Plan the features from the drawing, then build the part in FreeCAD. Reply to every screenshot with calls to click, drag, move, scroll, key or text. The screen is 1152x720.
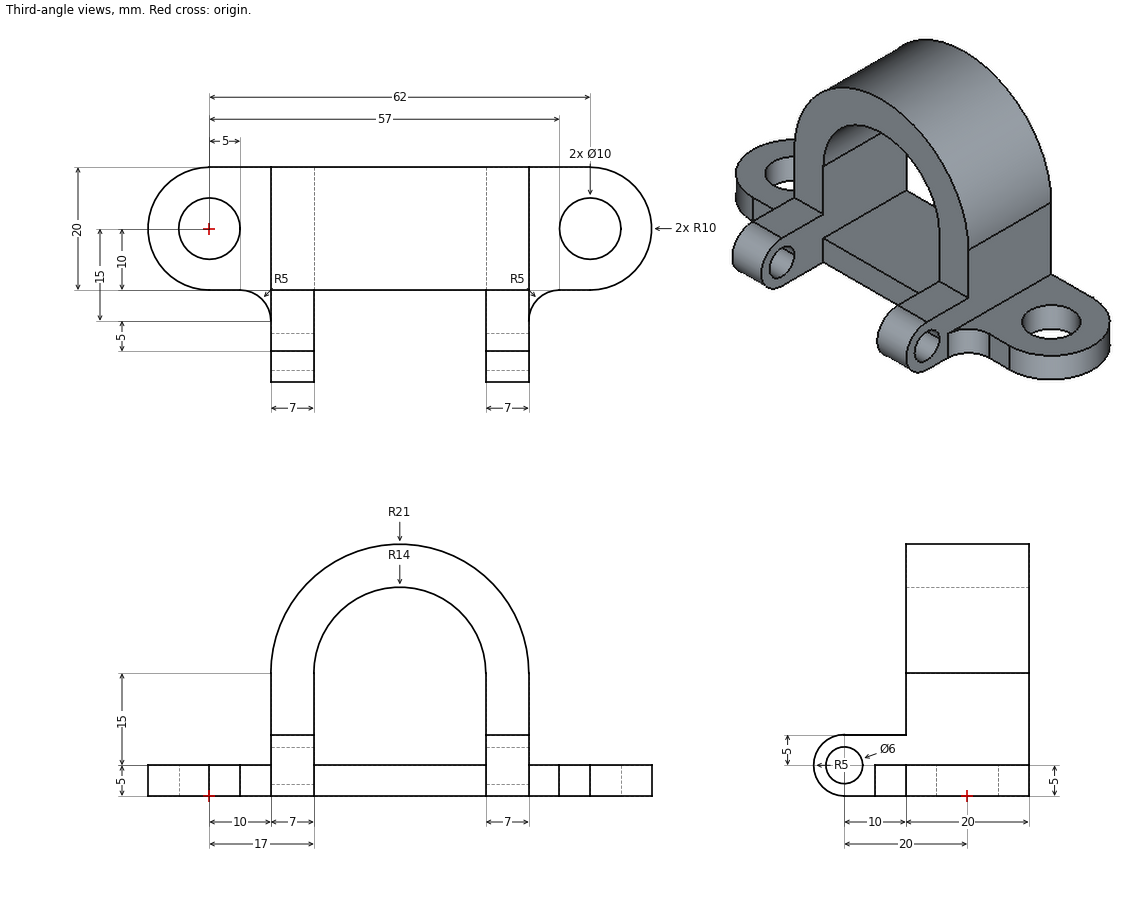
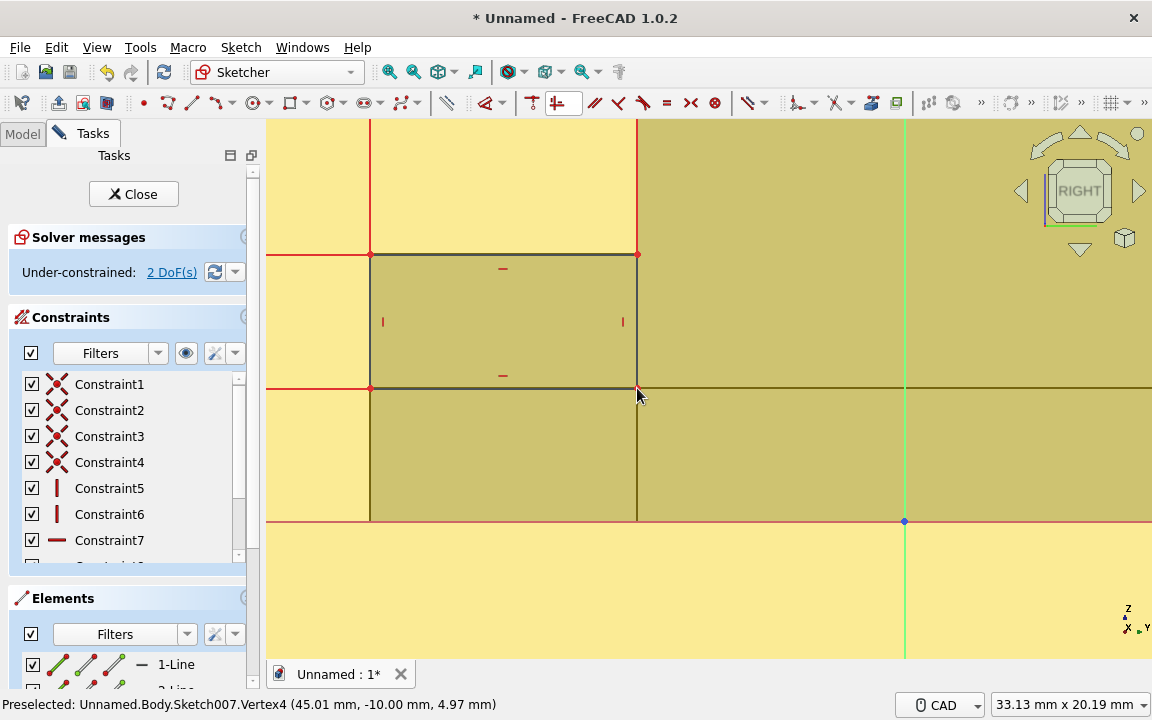
click(486, 104)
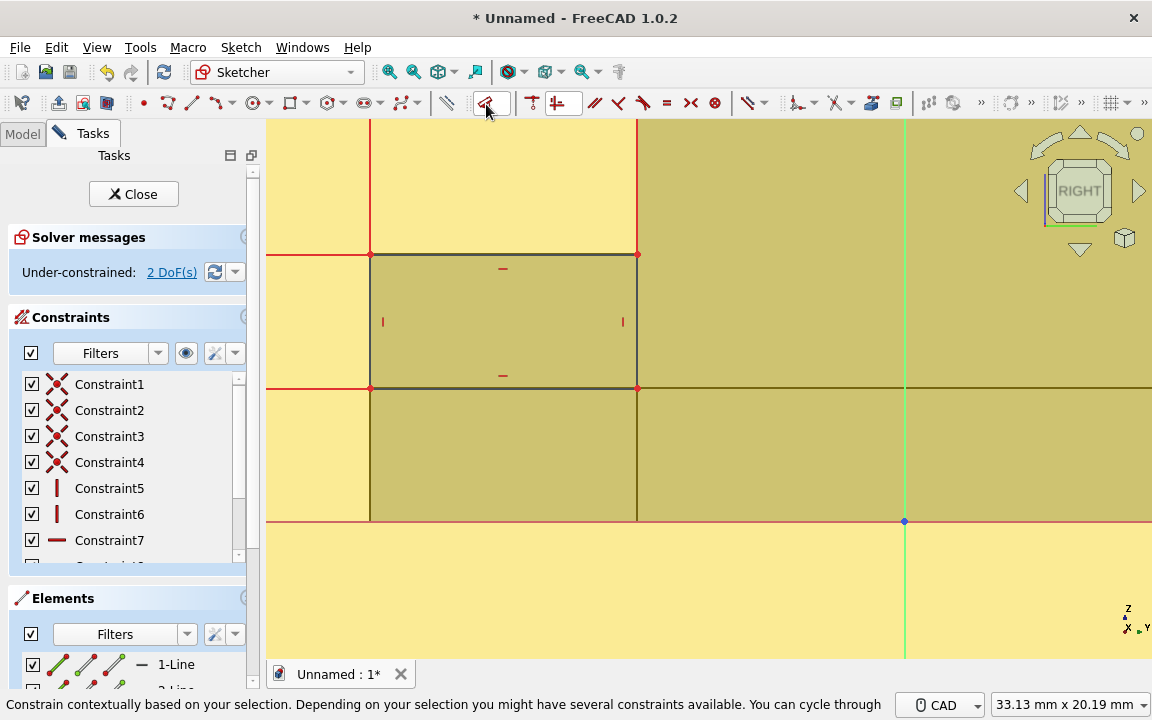
click(370, 389)
click(939, 455)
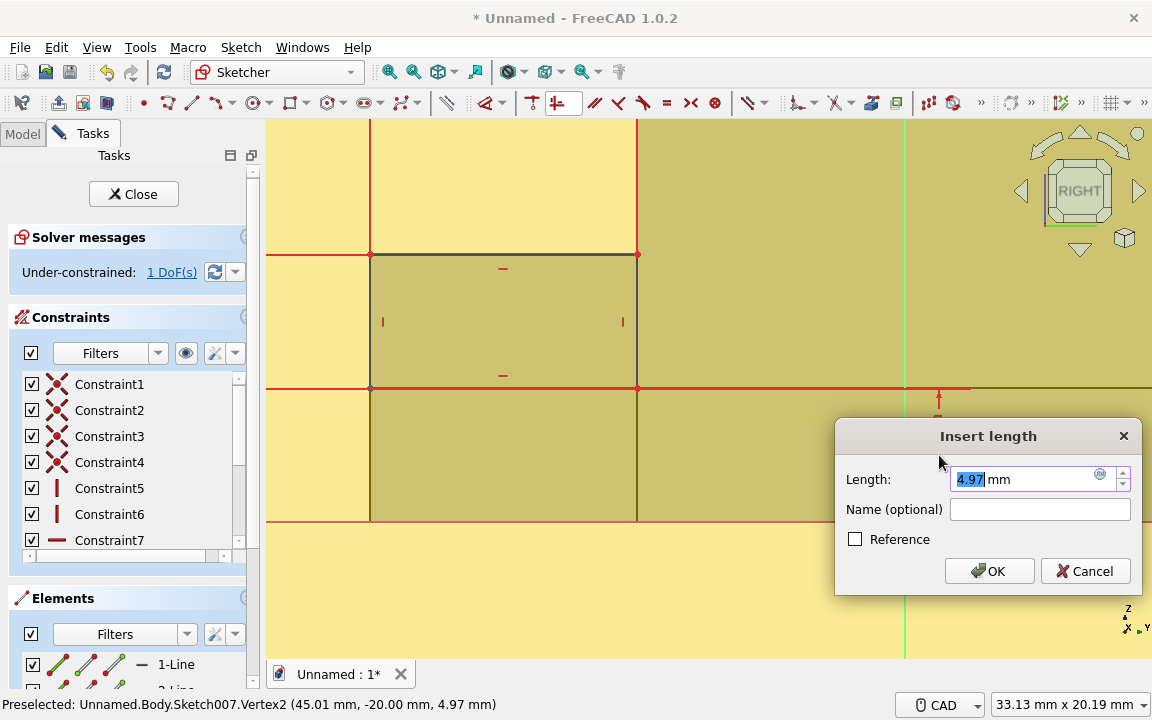
text(5)
key(Return)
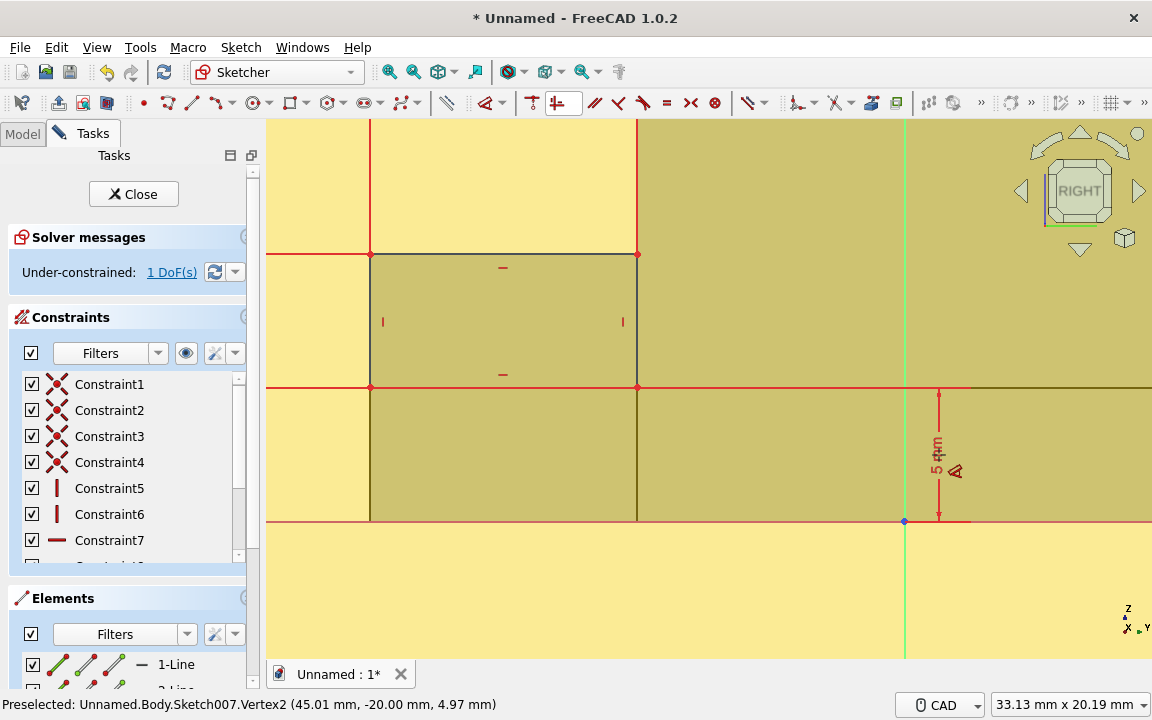
click(370, 254)
click(637, 556)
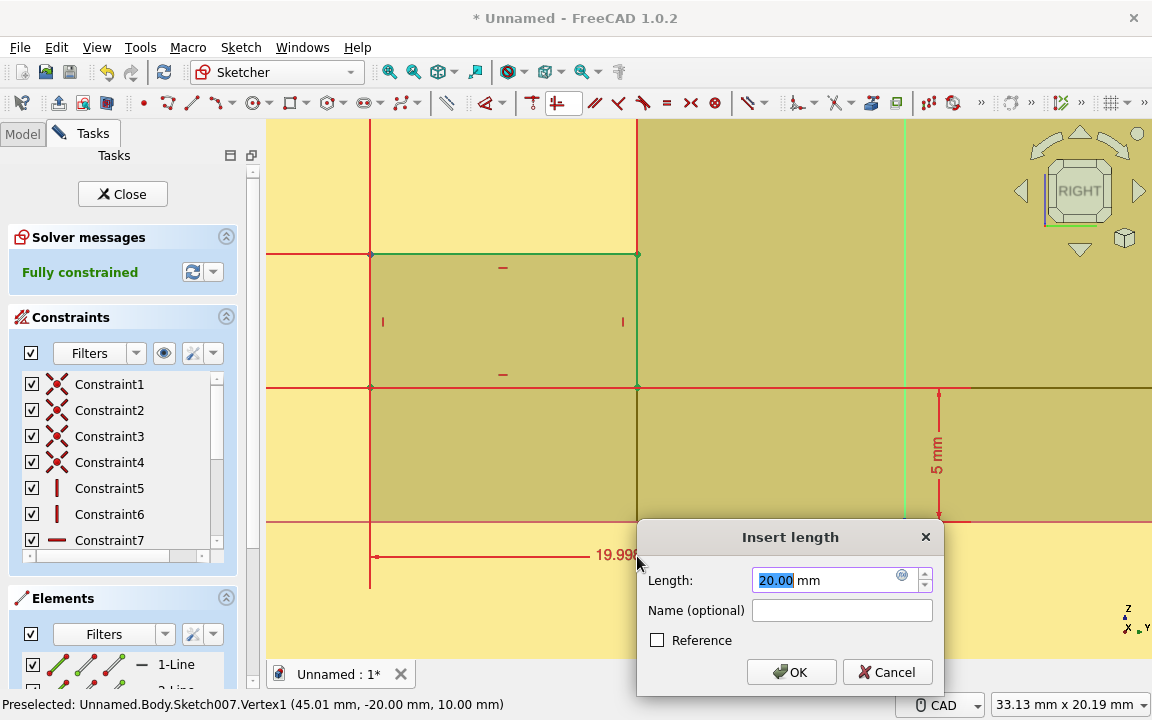
text(20)
key(Return)
key(Escape)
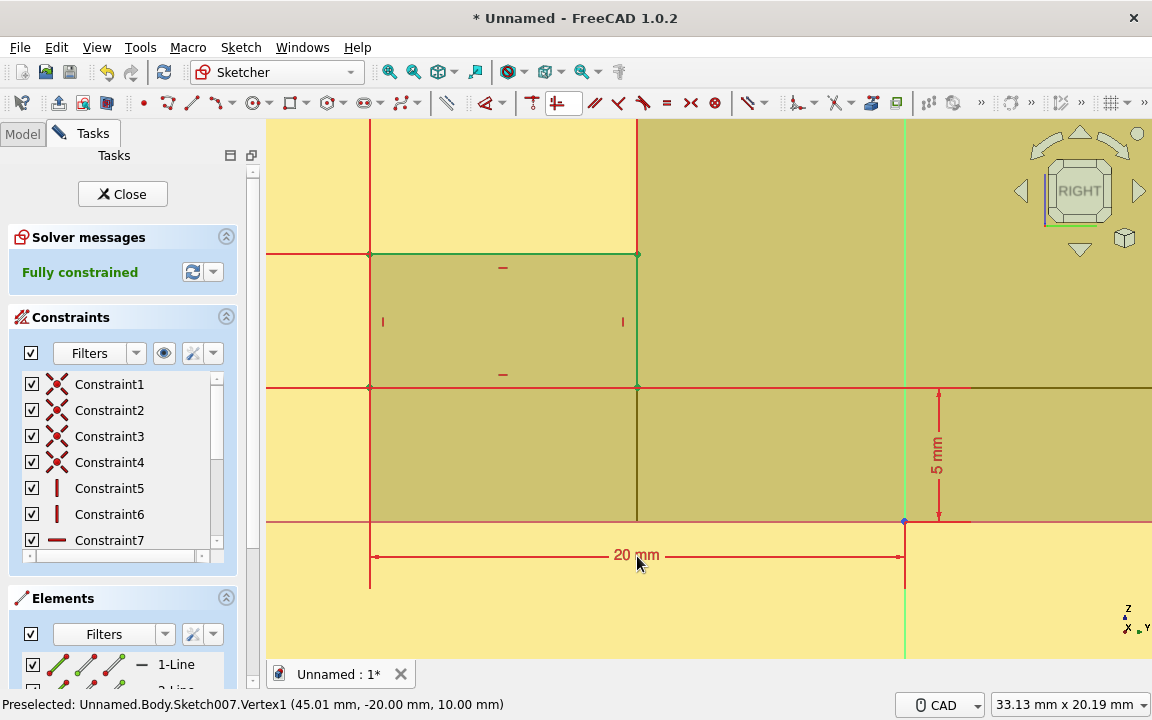
click(123, 194)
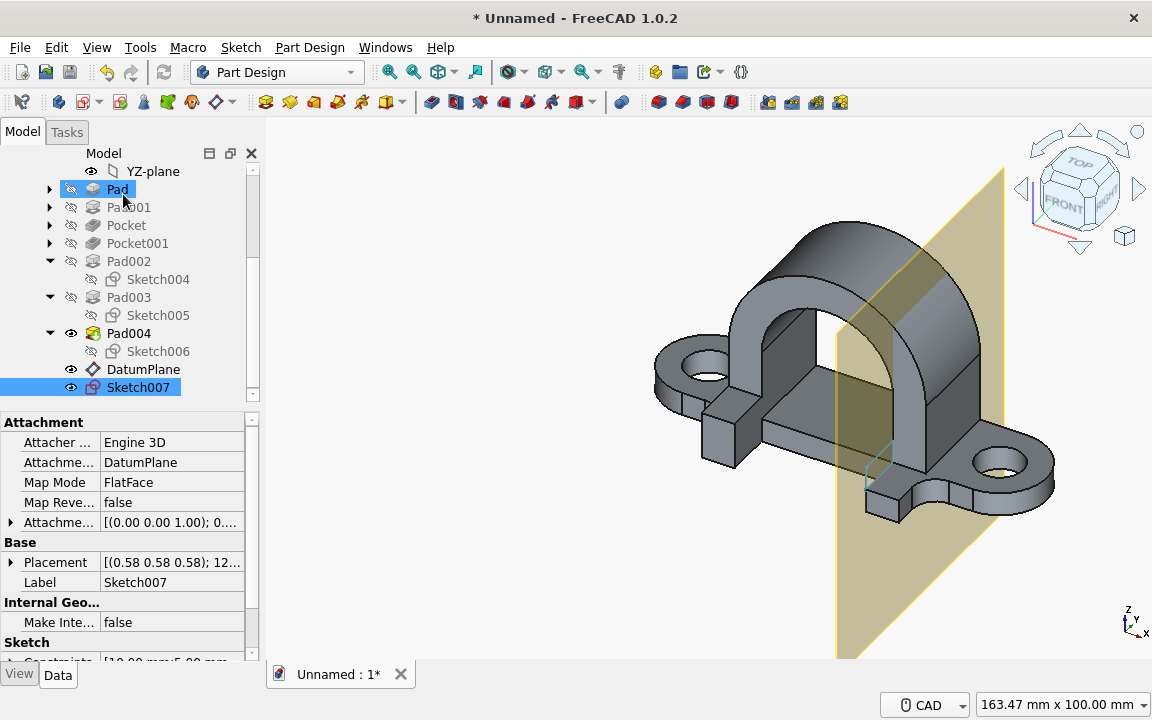
click(266, 102)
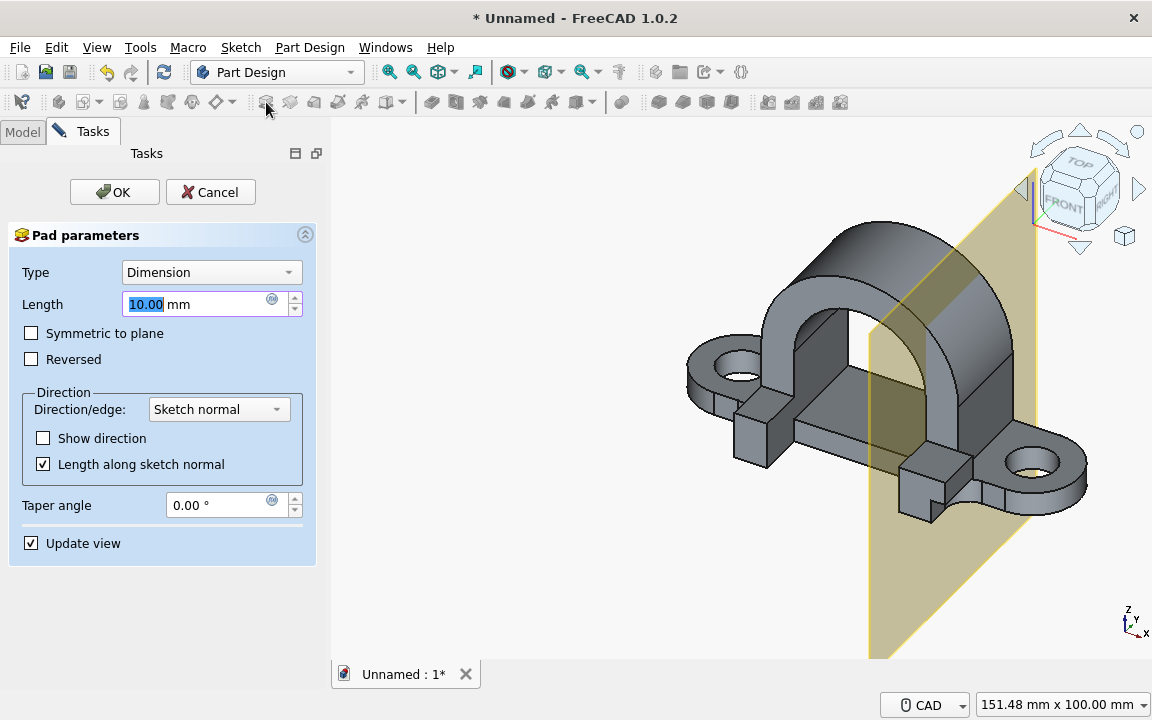
text(7)
key(Tab)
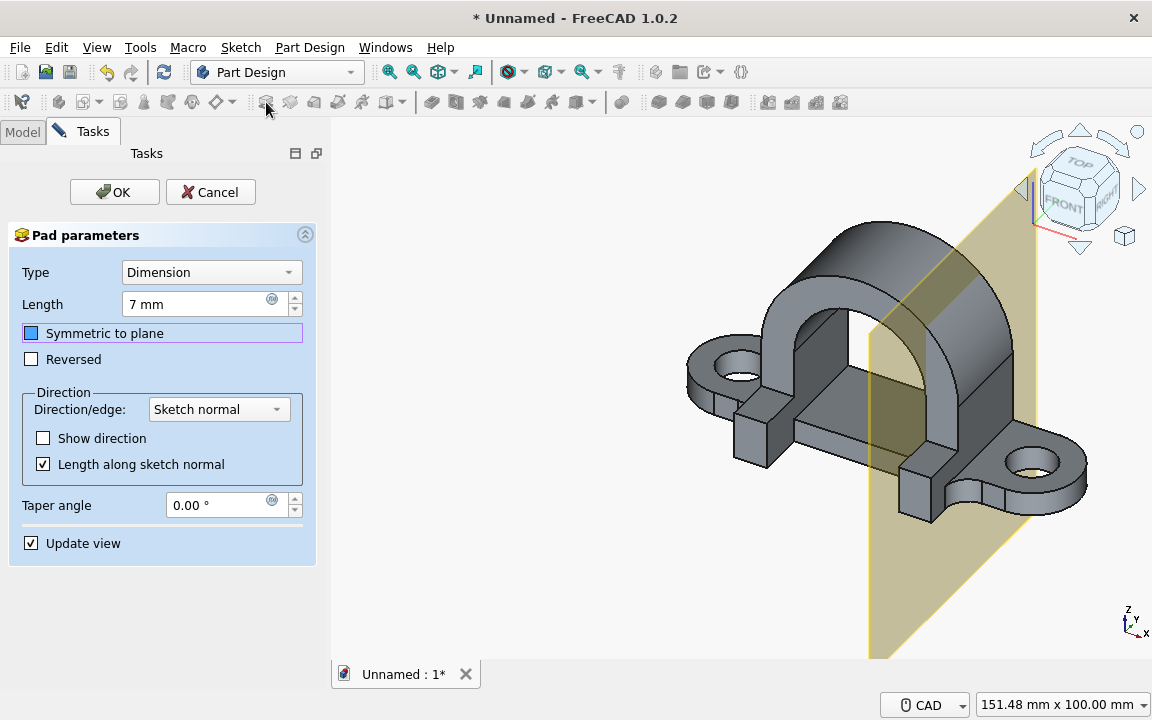
click(115, 192)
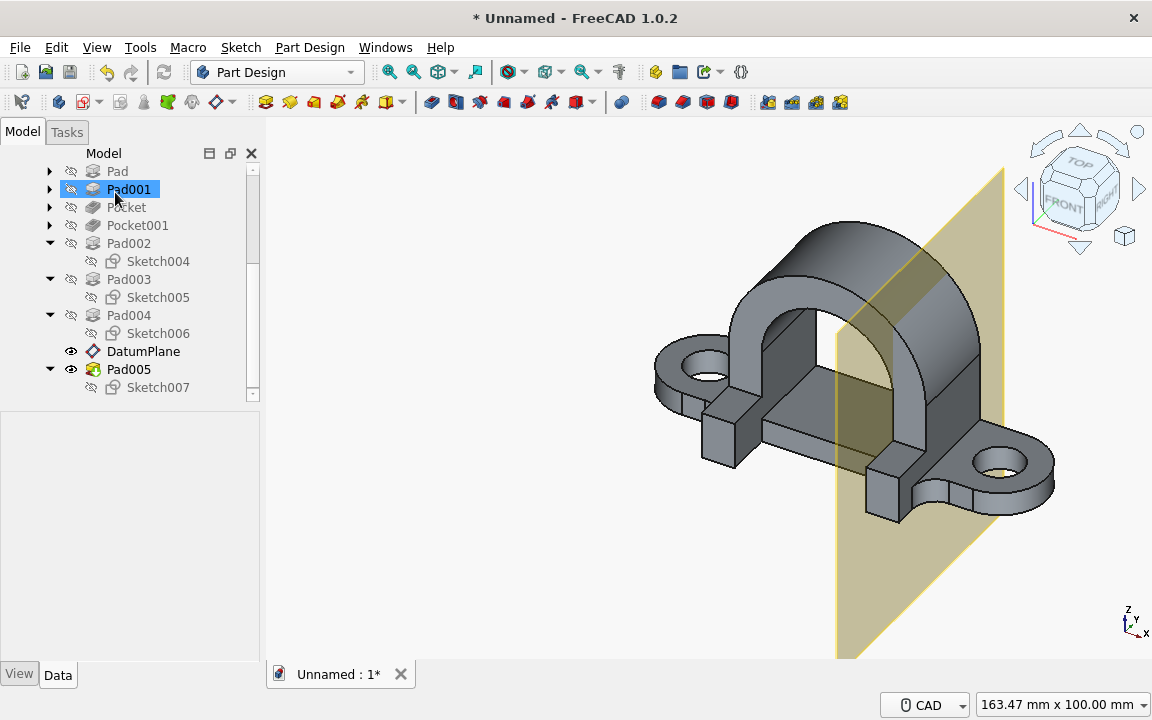
click(116, 351)
key(space)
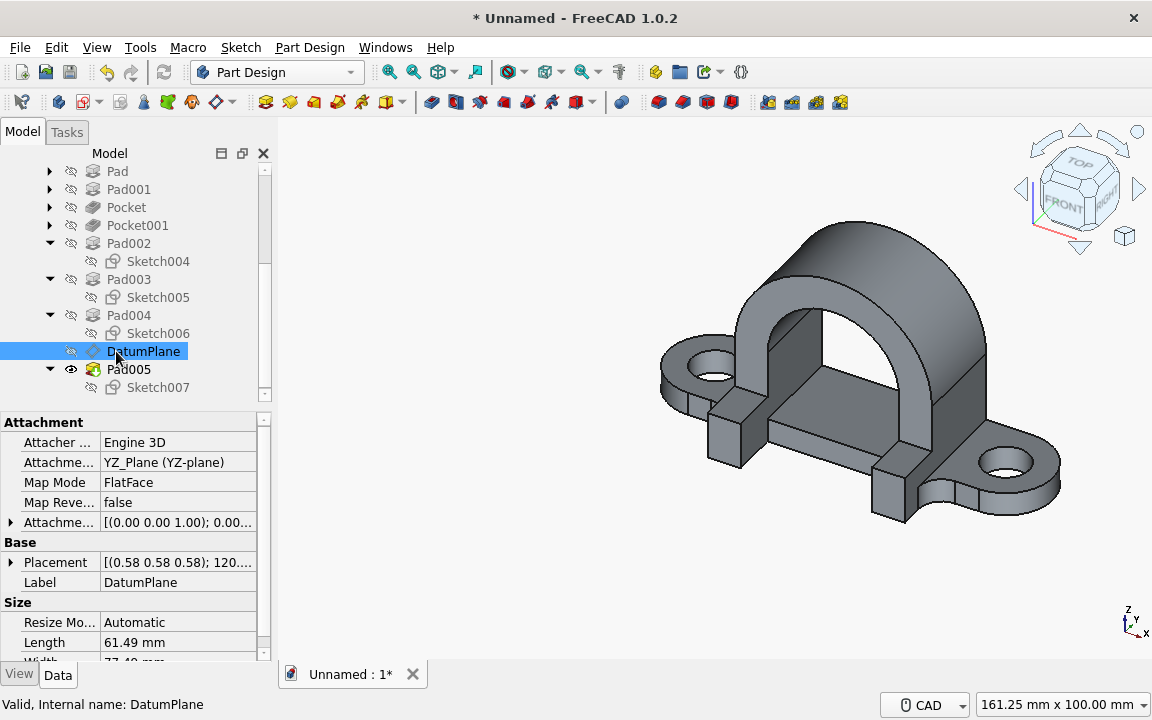
key(6)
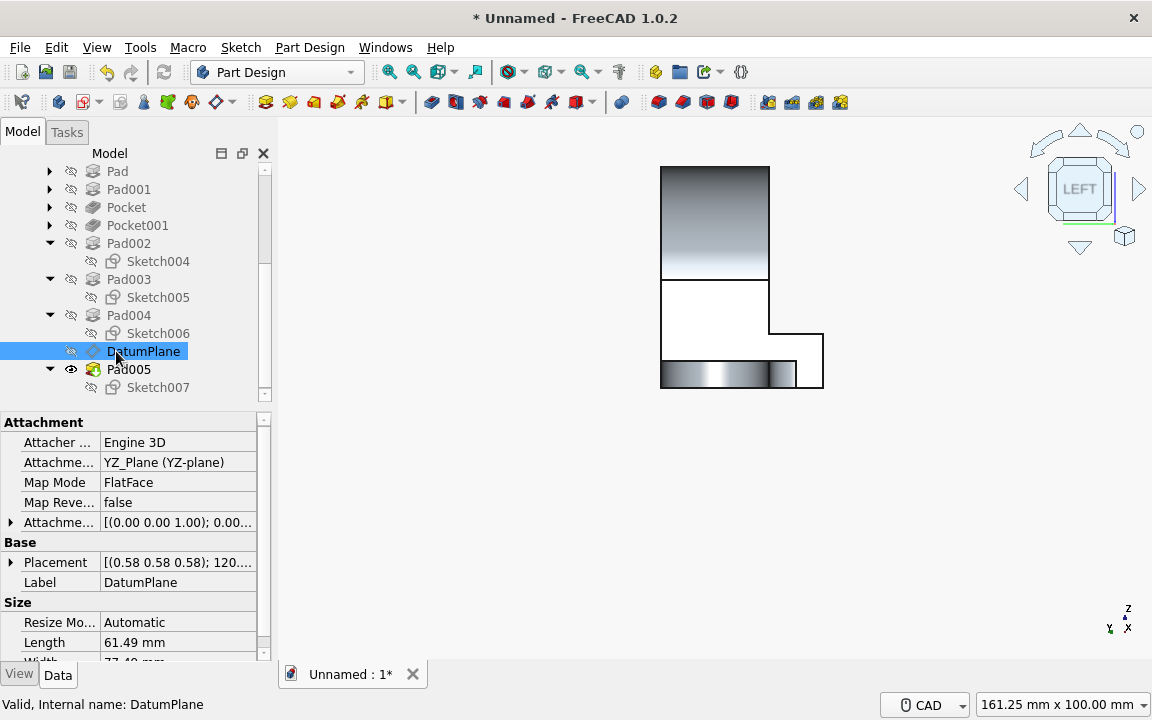
click(390, 72)